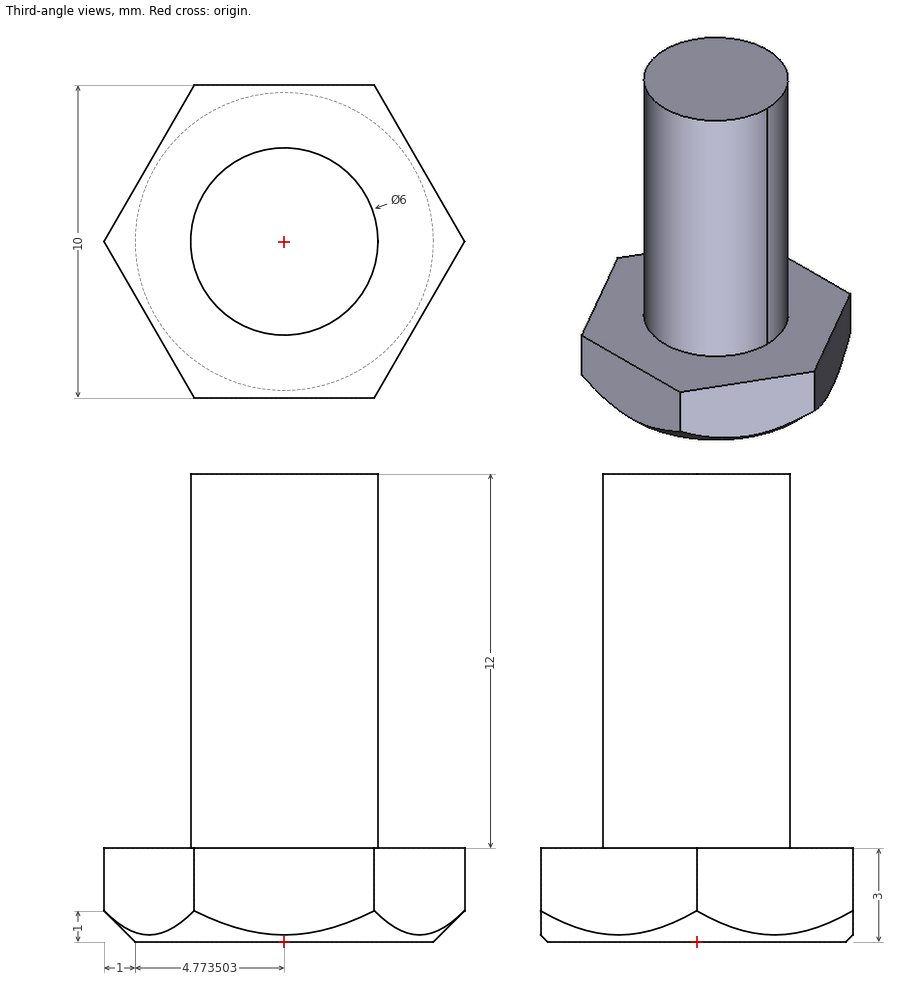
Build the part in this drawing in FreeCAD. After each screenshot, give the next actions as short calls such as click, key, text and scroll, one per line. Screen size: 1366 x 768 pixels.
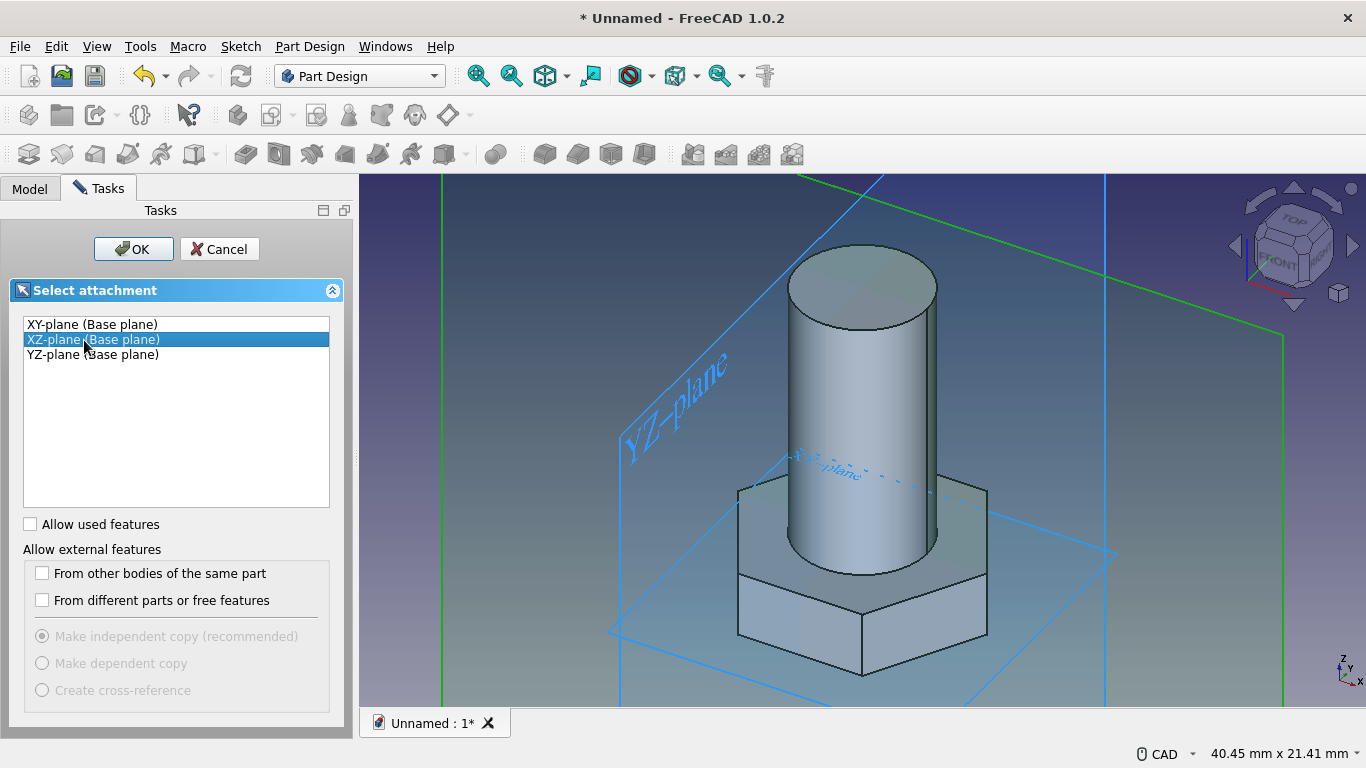
click(134, 249)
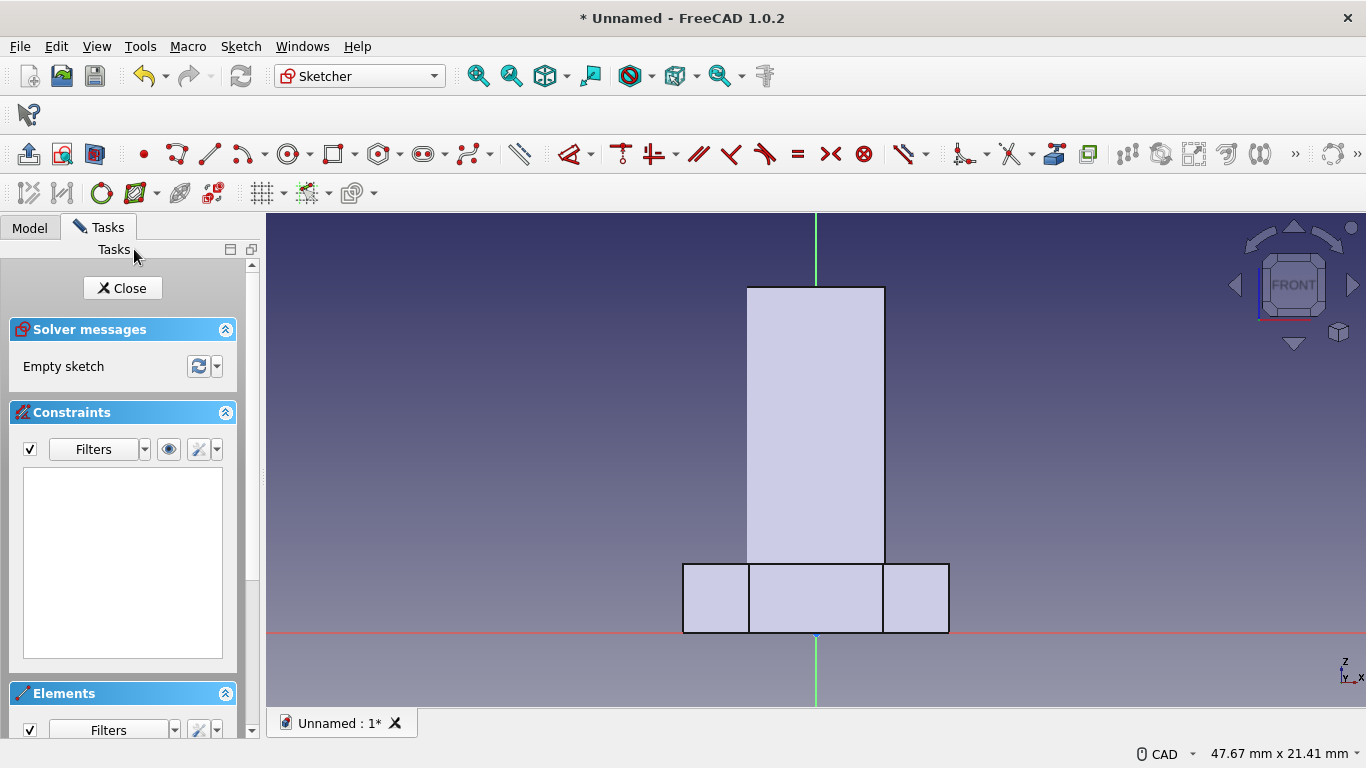
click(95, 154)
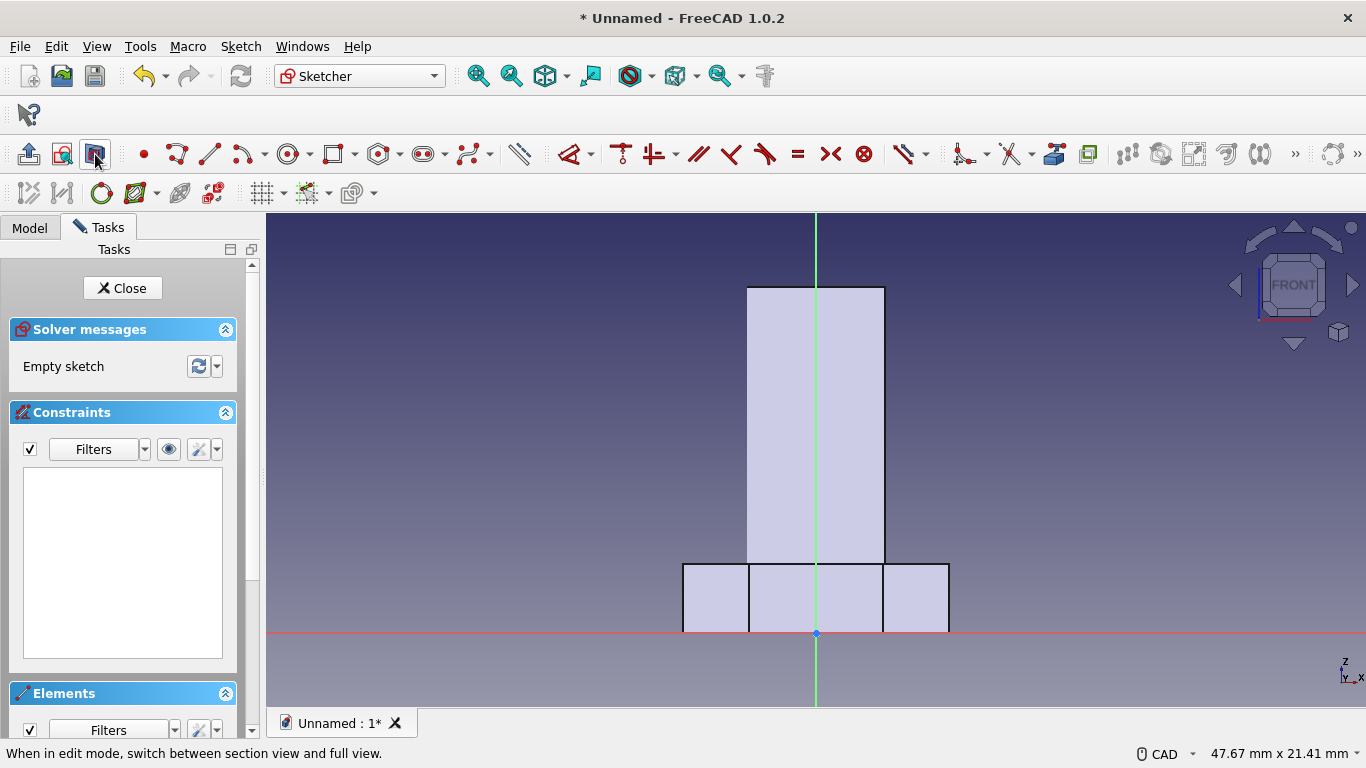
scroll(690, 634, up, 13)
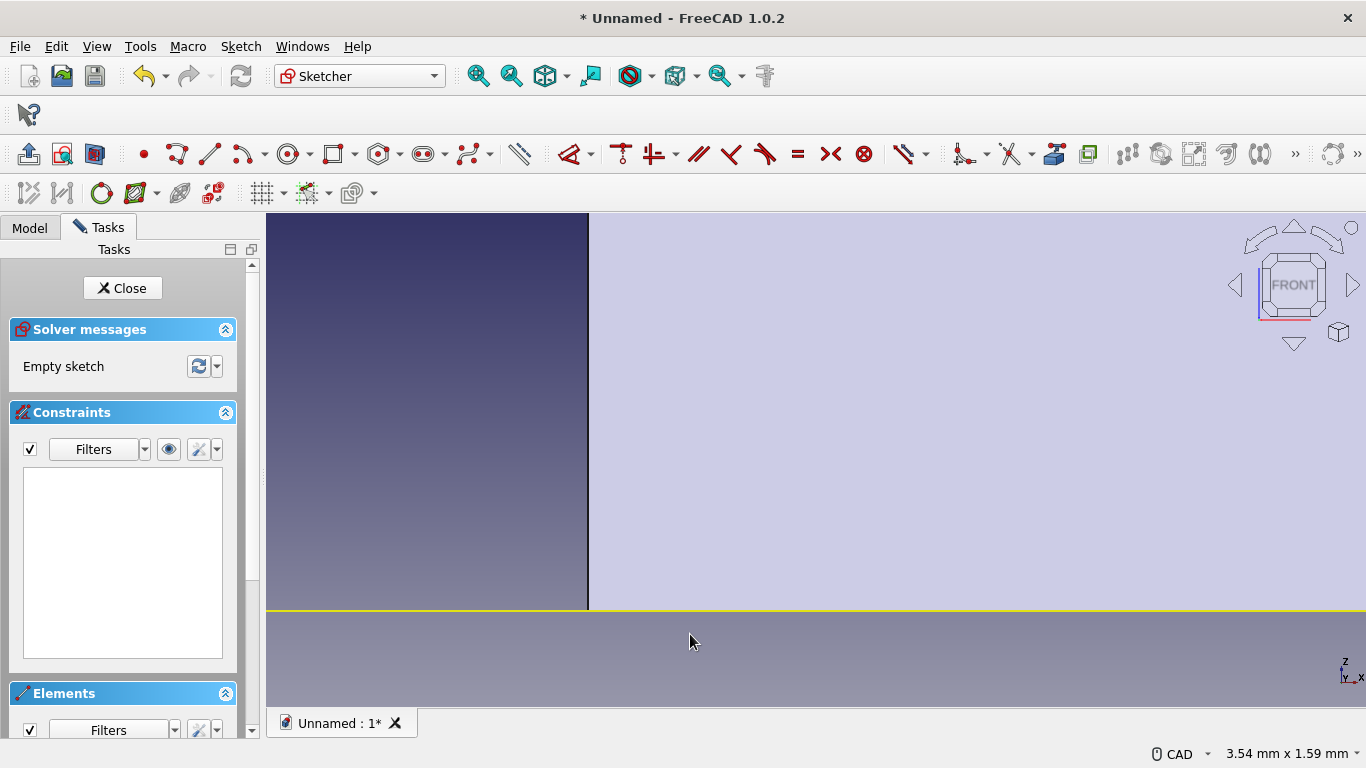
click(177, 154)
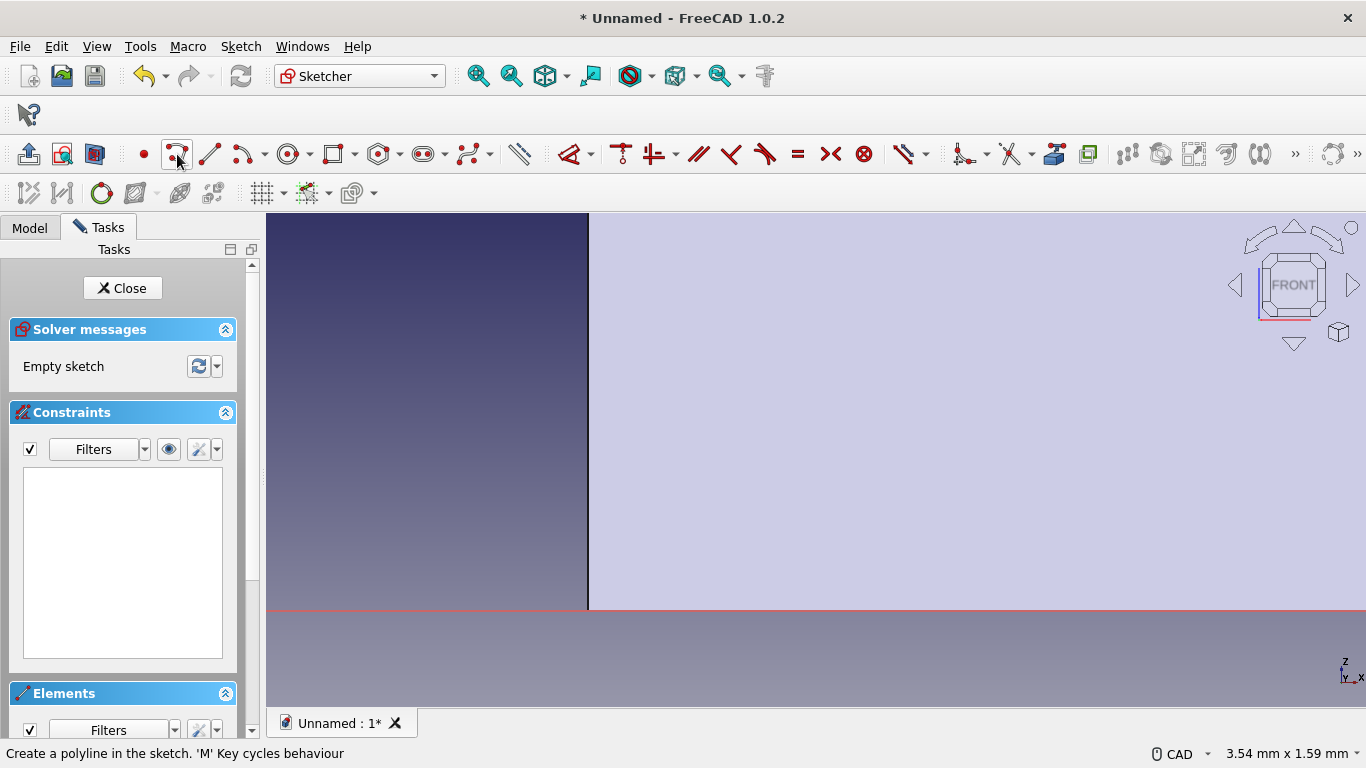
click(899, 611)
click(588, 602)
click(588, 300)
click(899, 611)
key(Escape)
key(Escape)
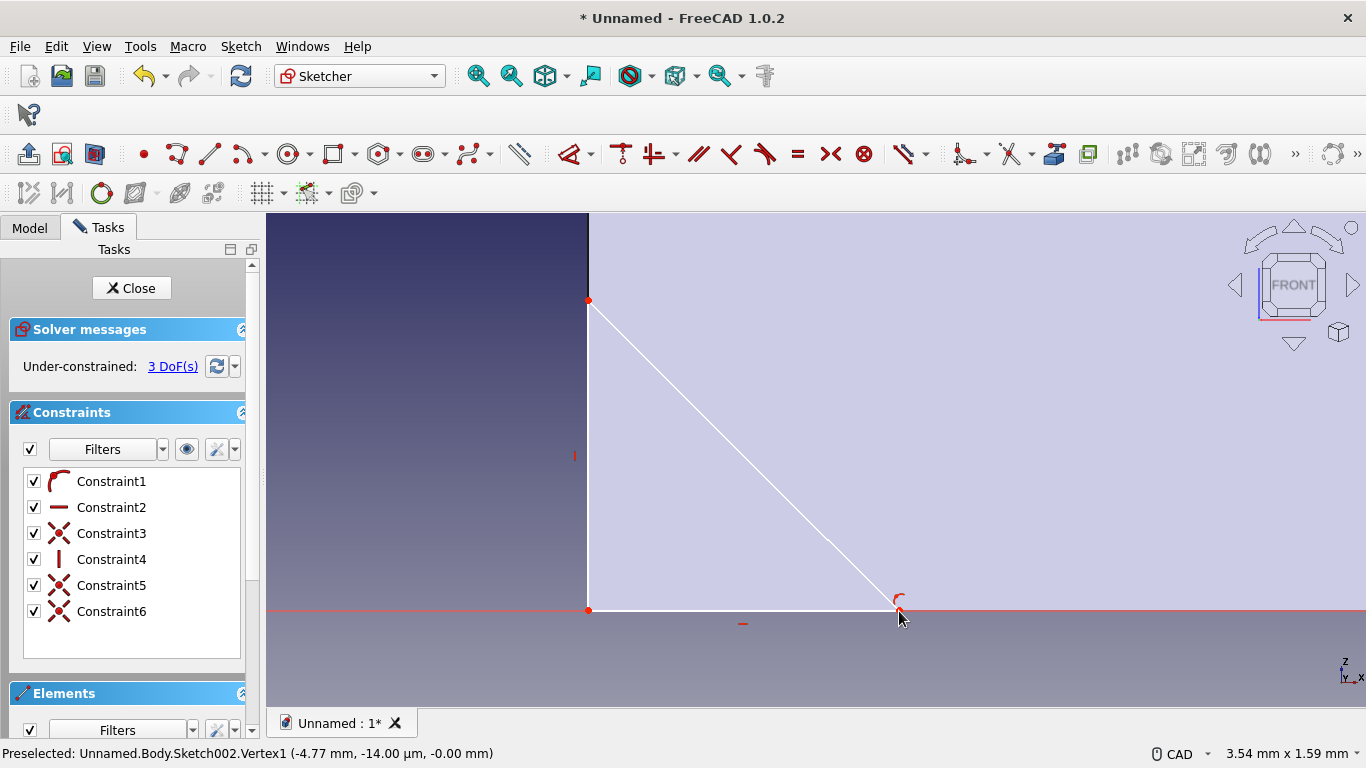
key(d)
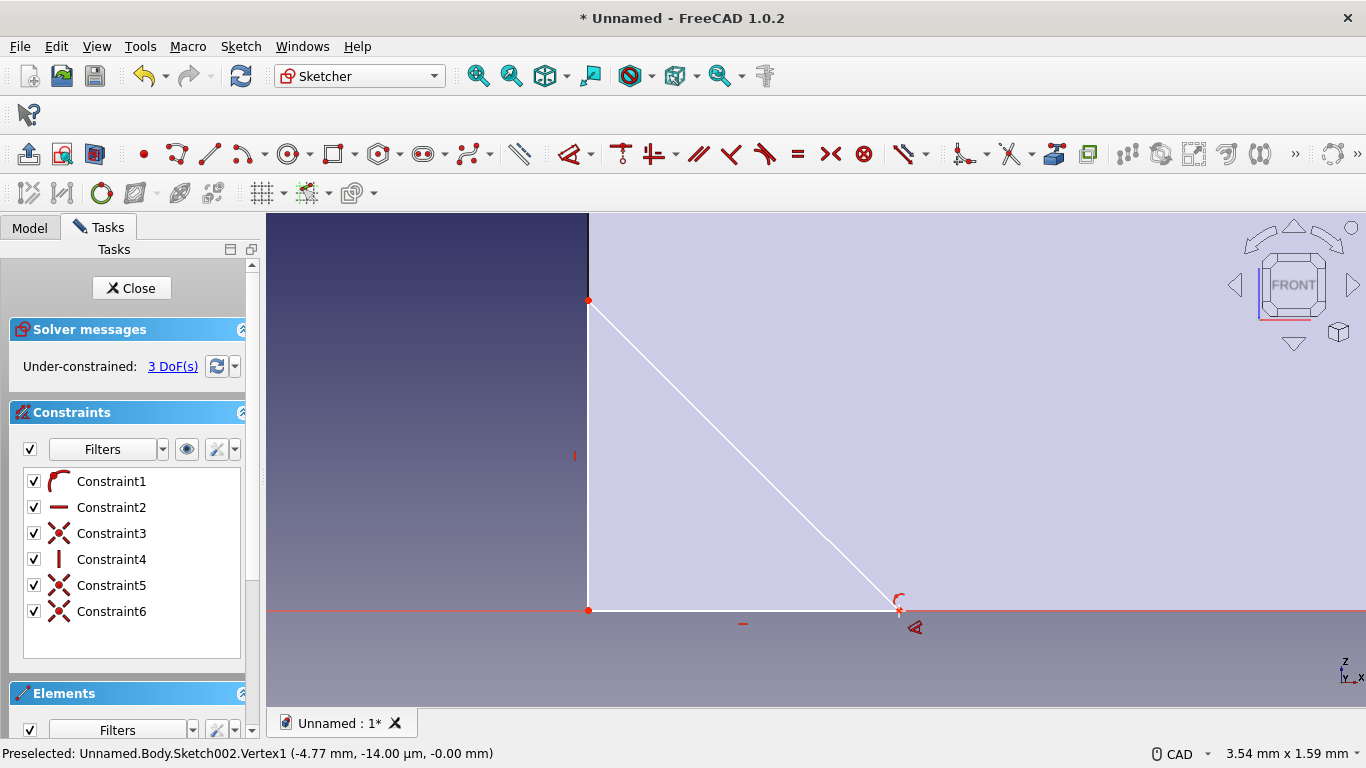
click(806, 611)
click(744, 645)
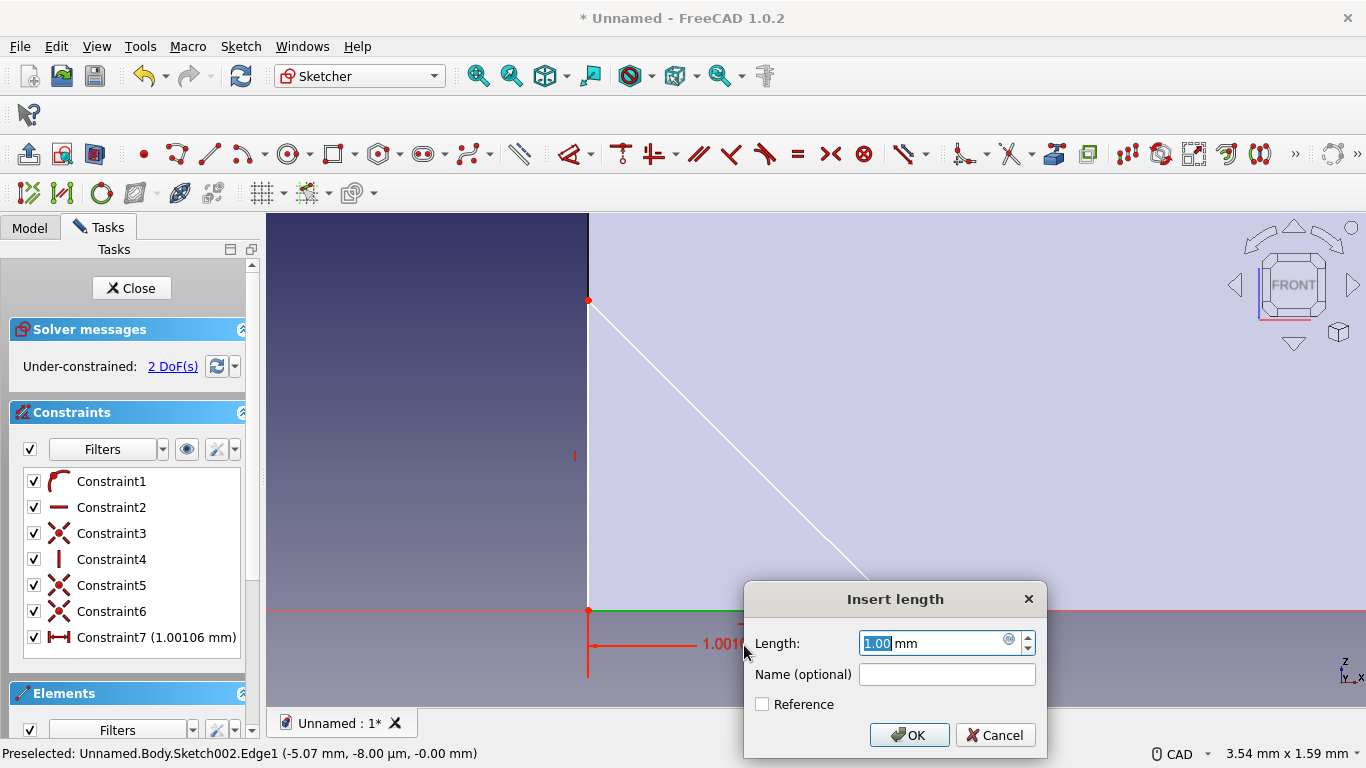
text(1)
key(Return)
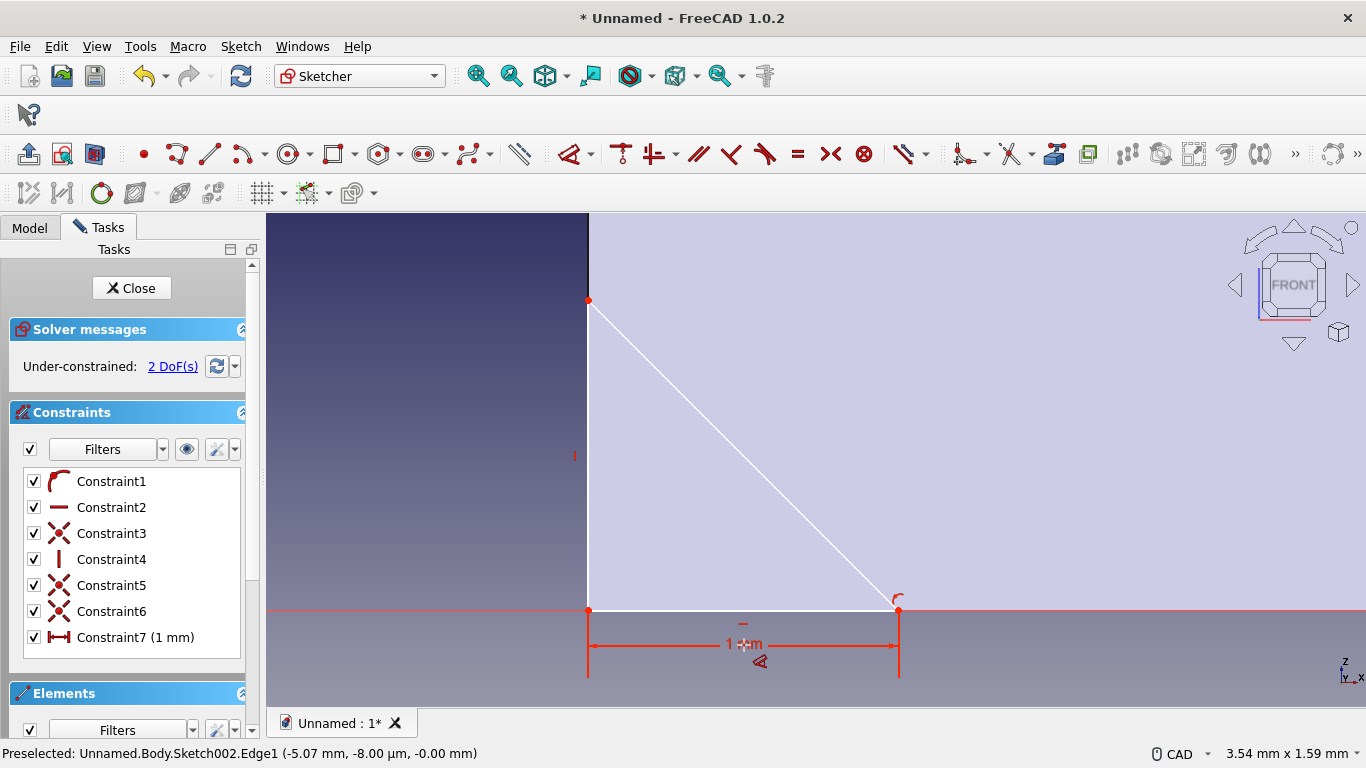
click(588, 518)
click(554, 456)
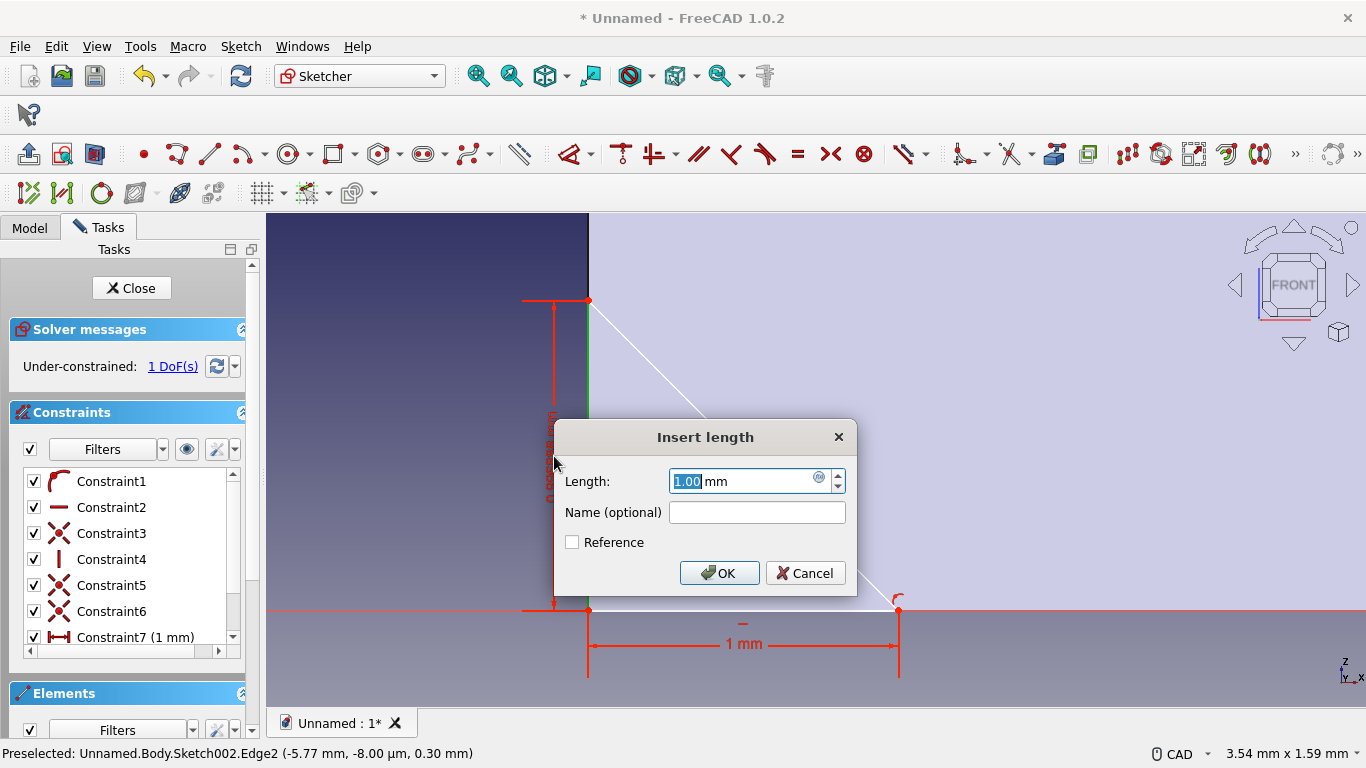
text(1)
key(Return)